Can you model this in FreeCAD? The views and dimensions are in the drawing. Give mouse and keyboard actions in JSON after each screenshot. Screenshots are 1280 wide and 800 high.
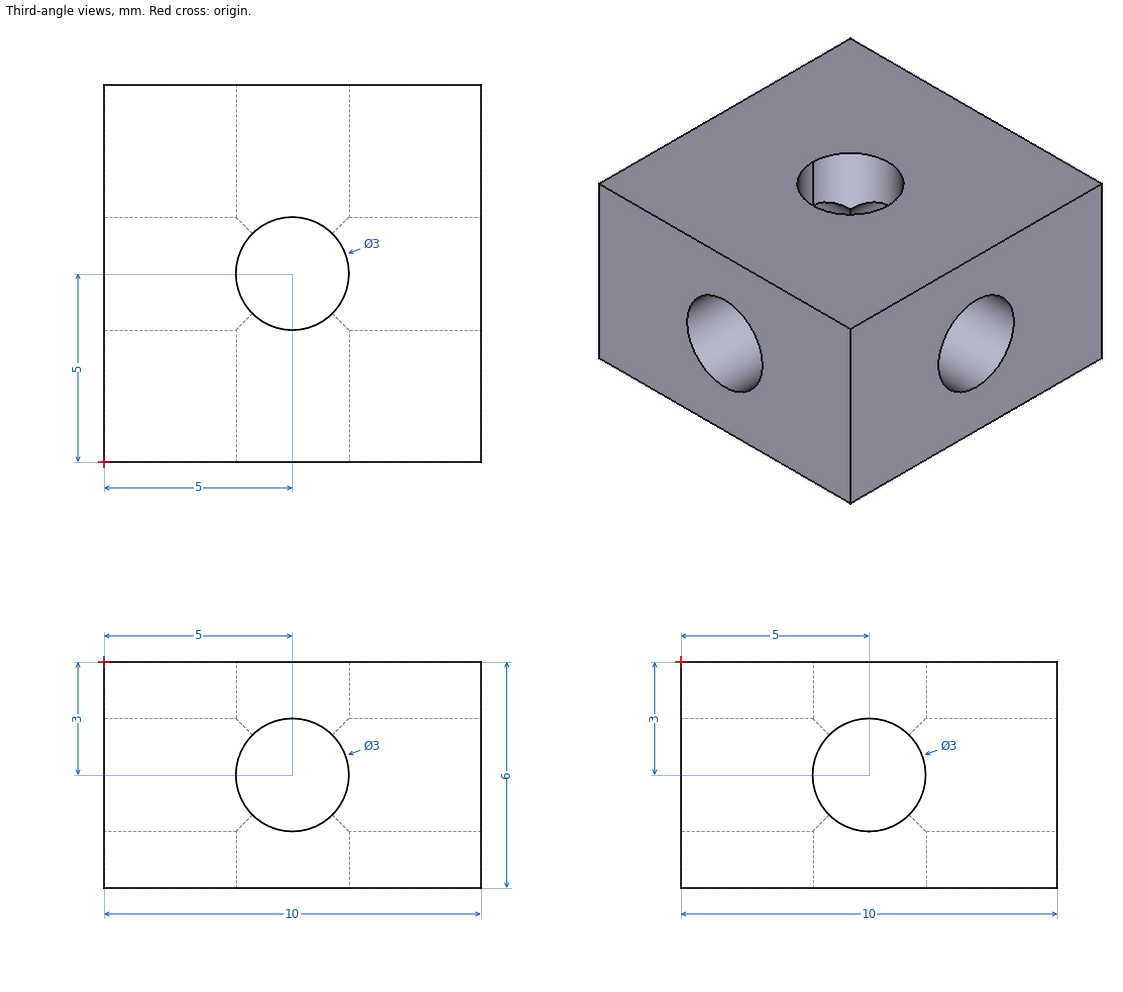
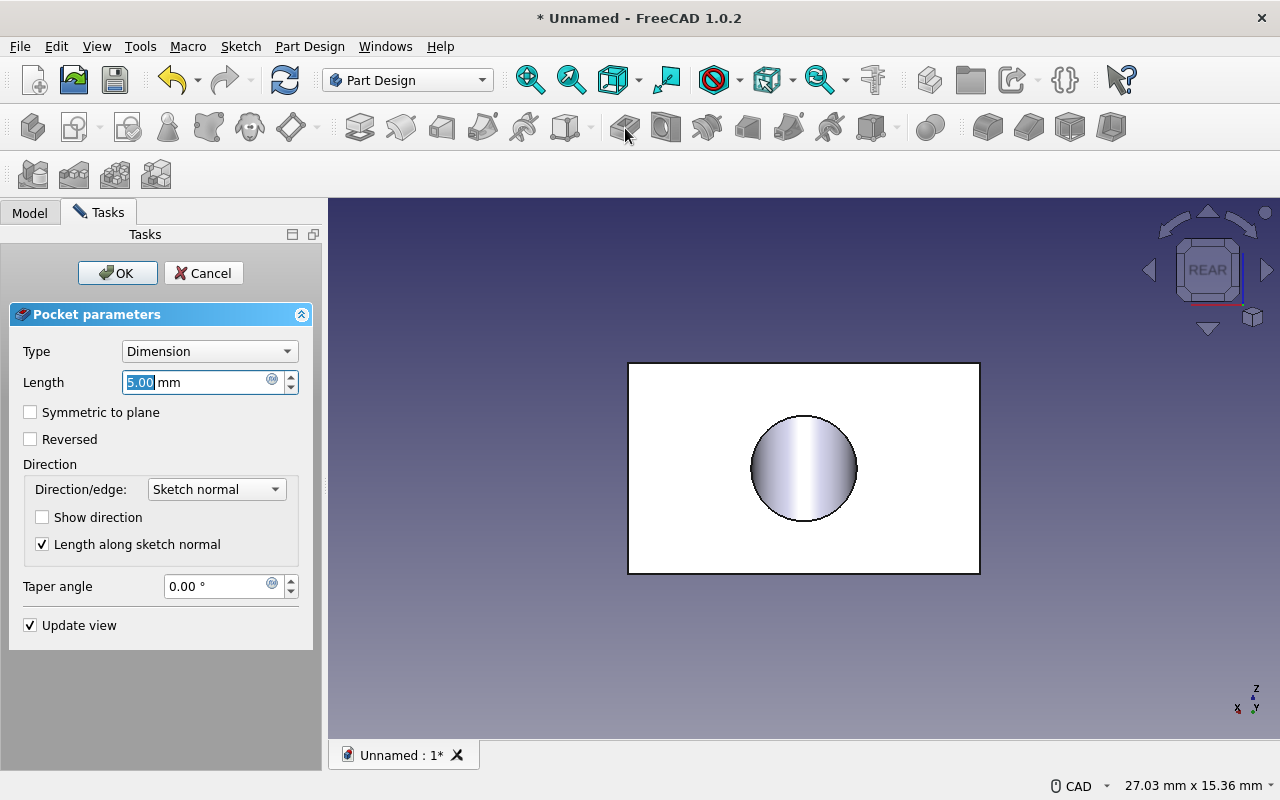
{"action": "left_click", "coordinate": [210, 352]}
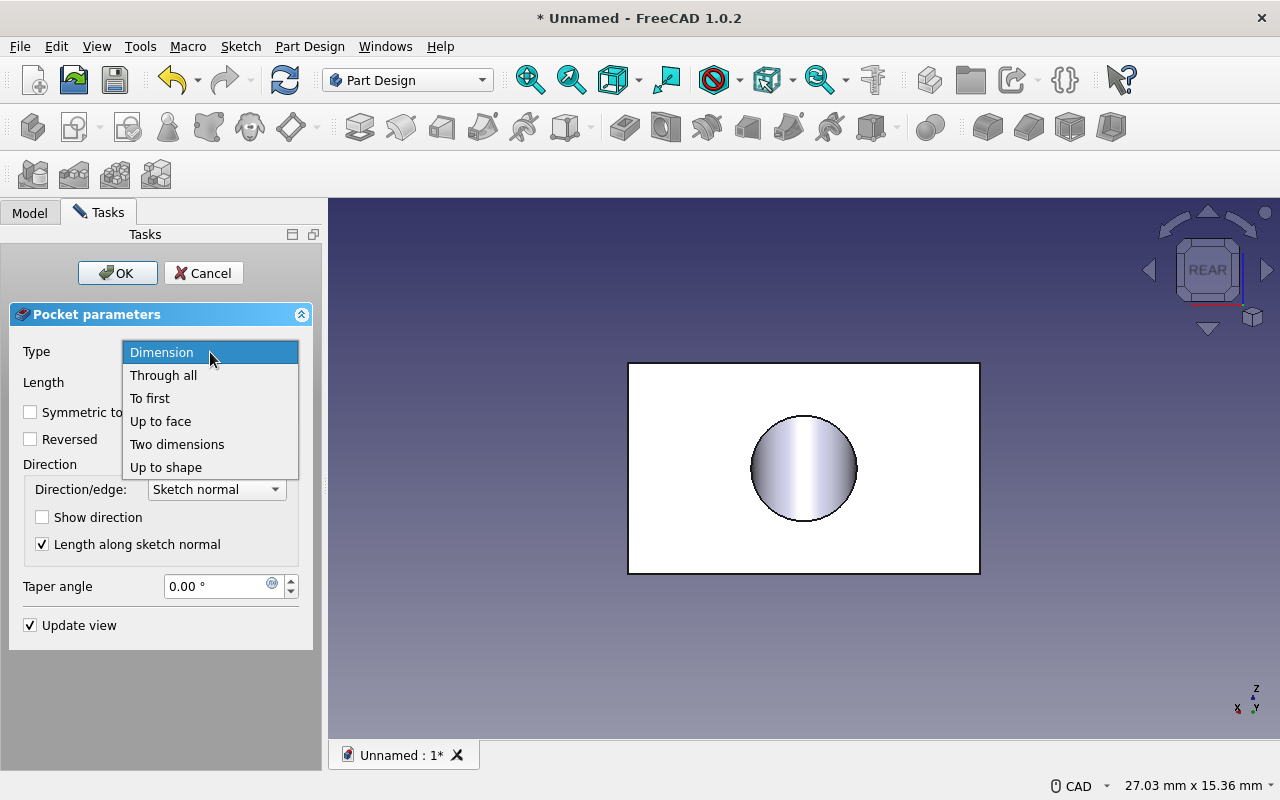
{"action": "left_click", "coordinate": [208, 376]}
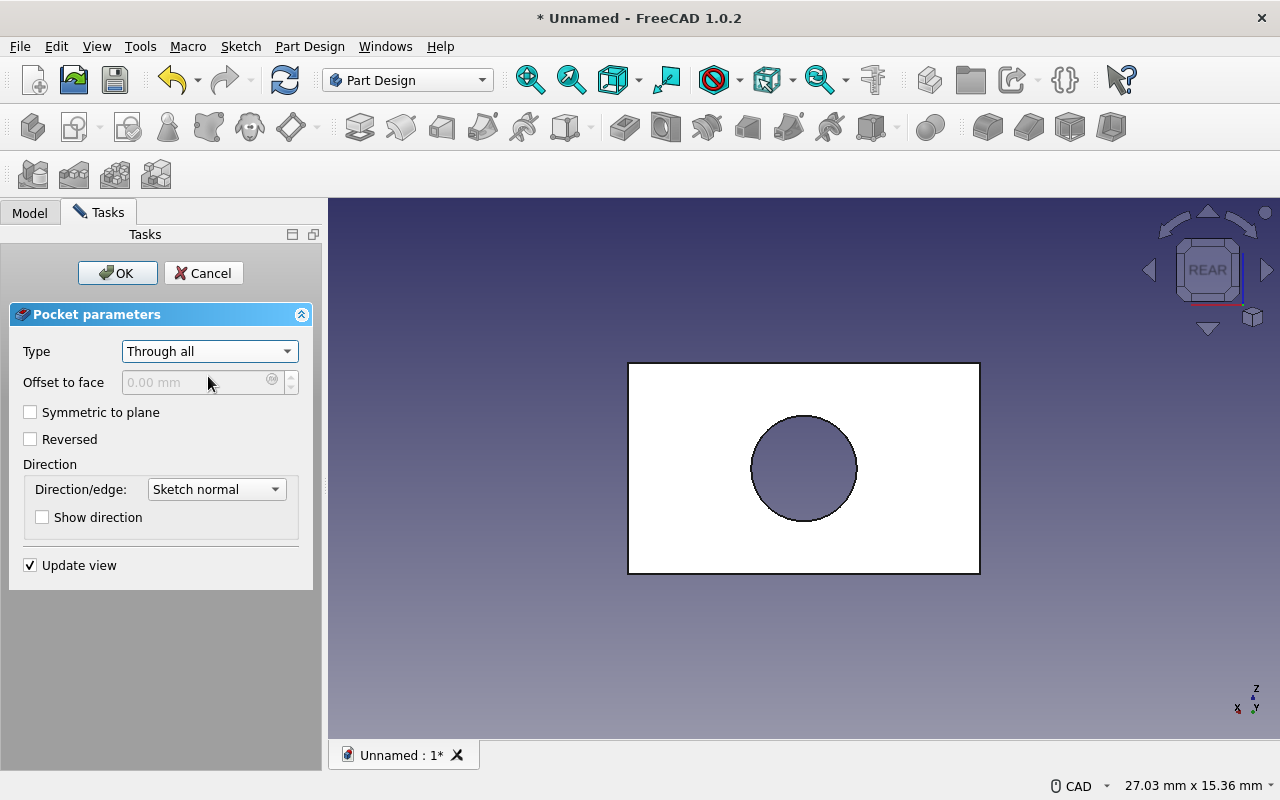
{"action": "left_click", "coordinate": [118, 273]}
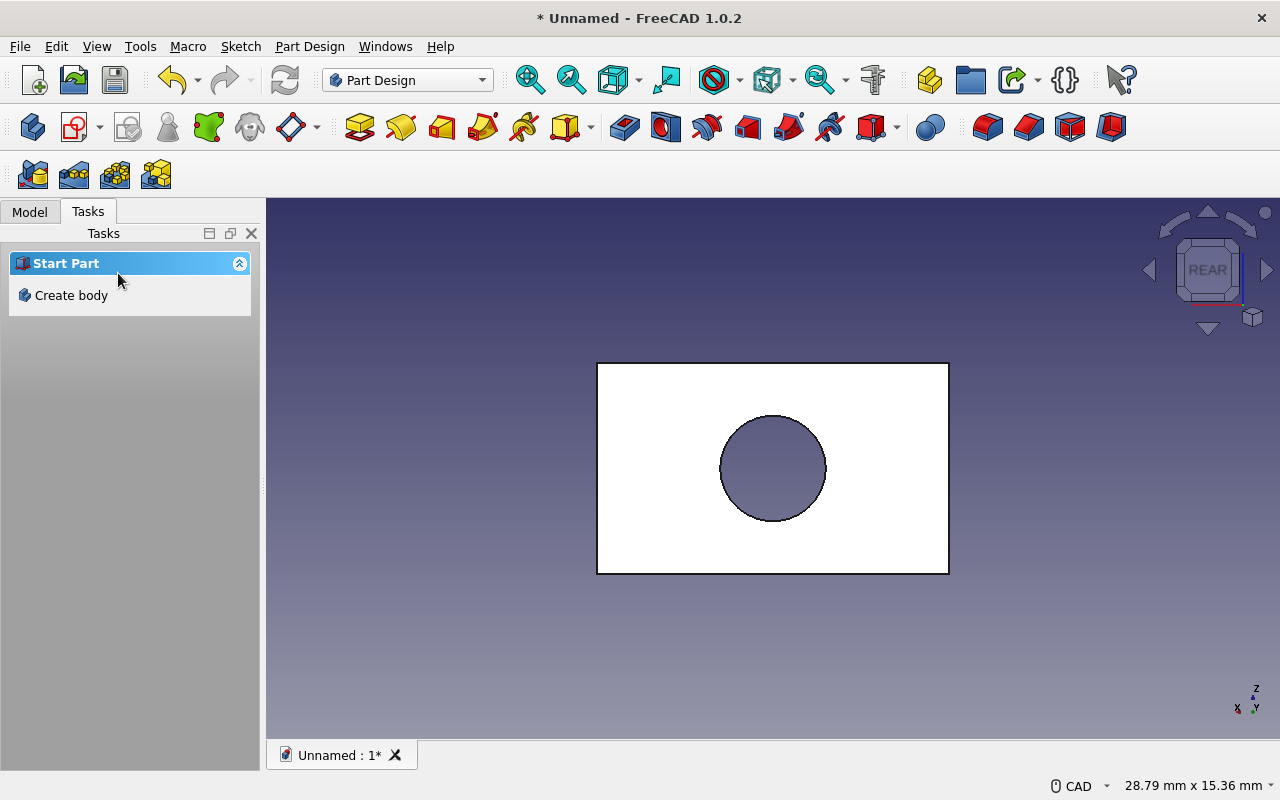
{"action": "left_click", "coordinate": [531, 80]}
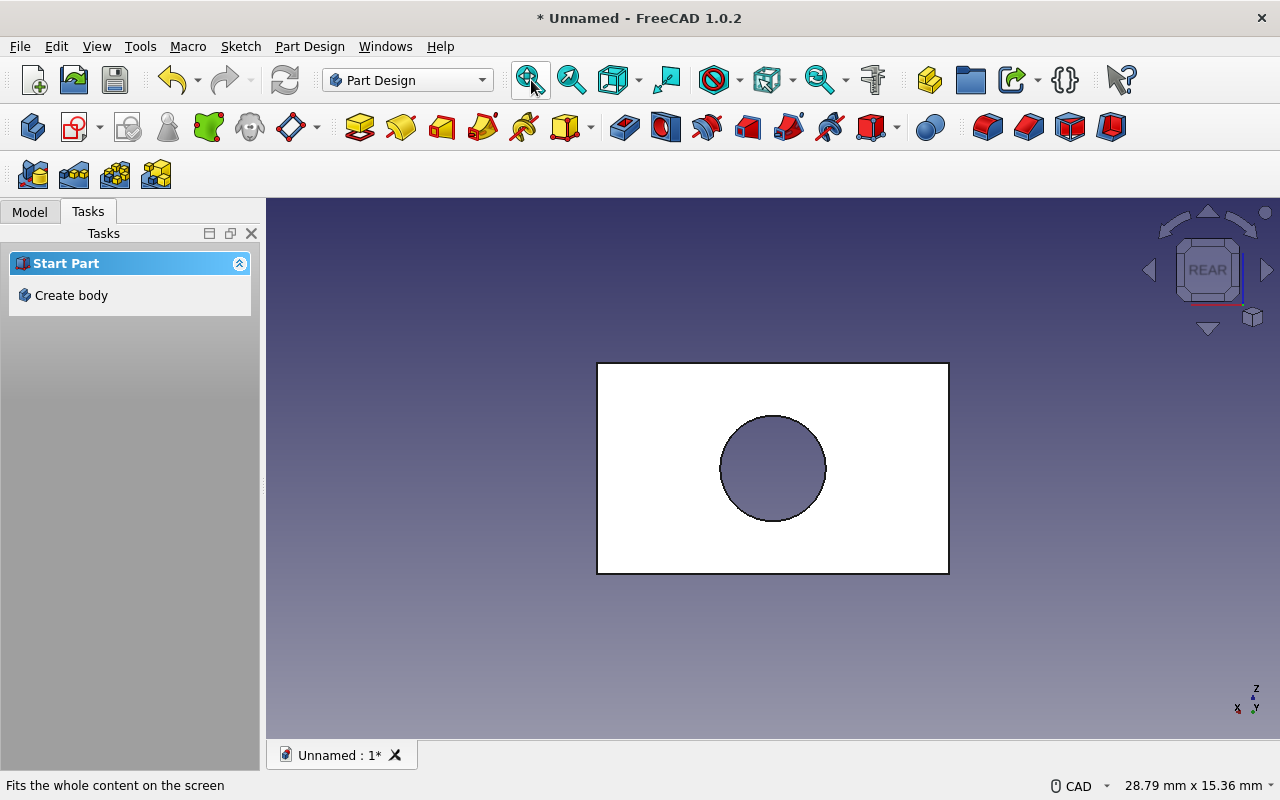
{"action": "key", "text": "0"}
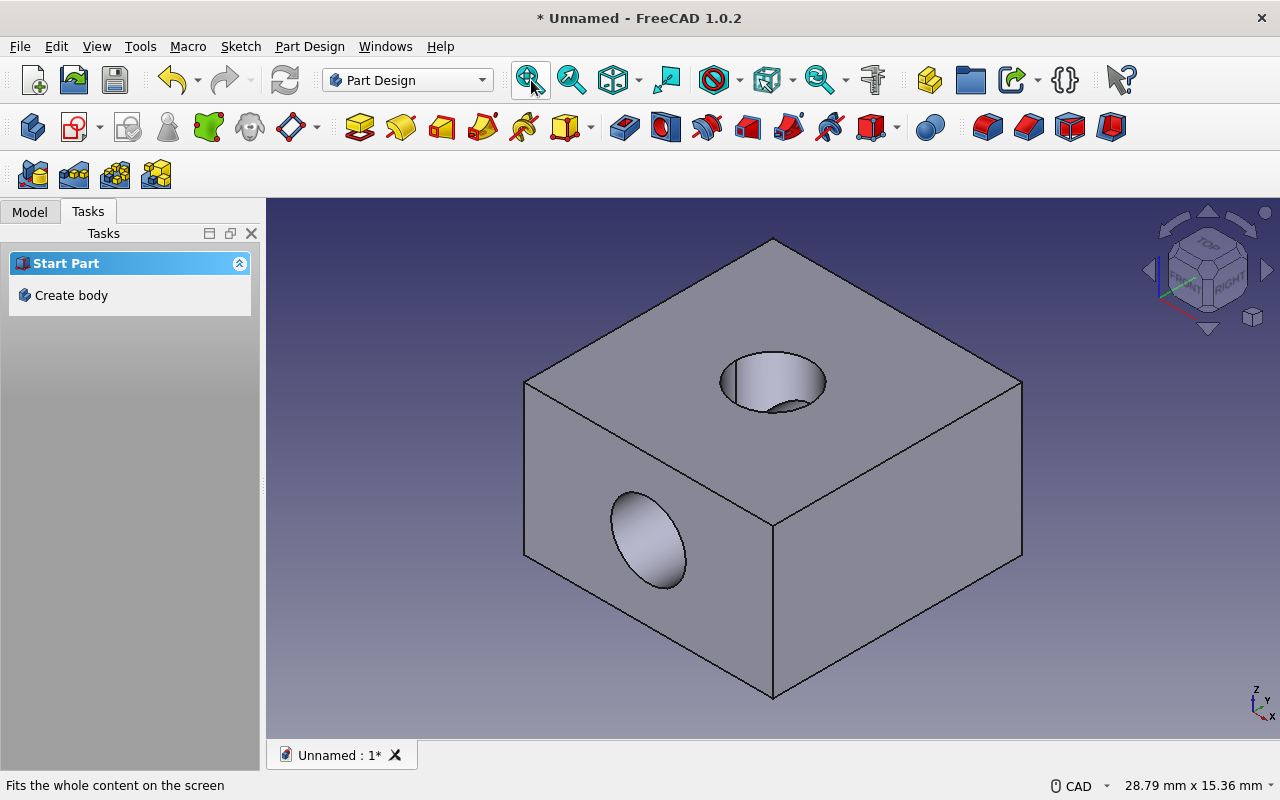
{"action": "left_click", "coordinate": [933, 519]}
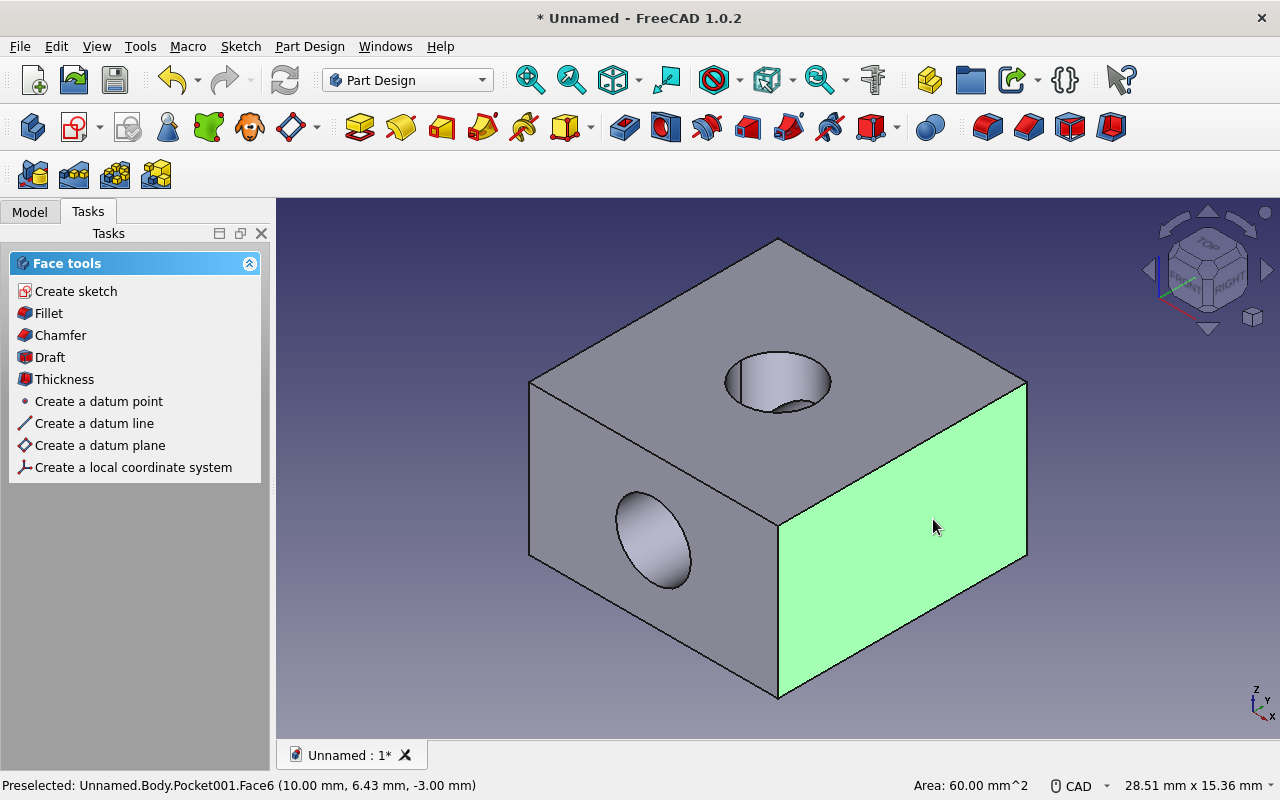
{"action": "left_click", "coordinate": [74, 128]}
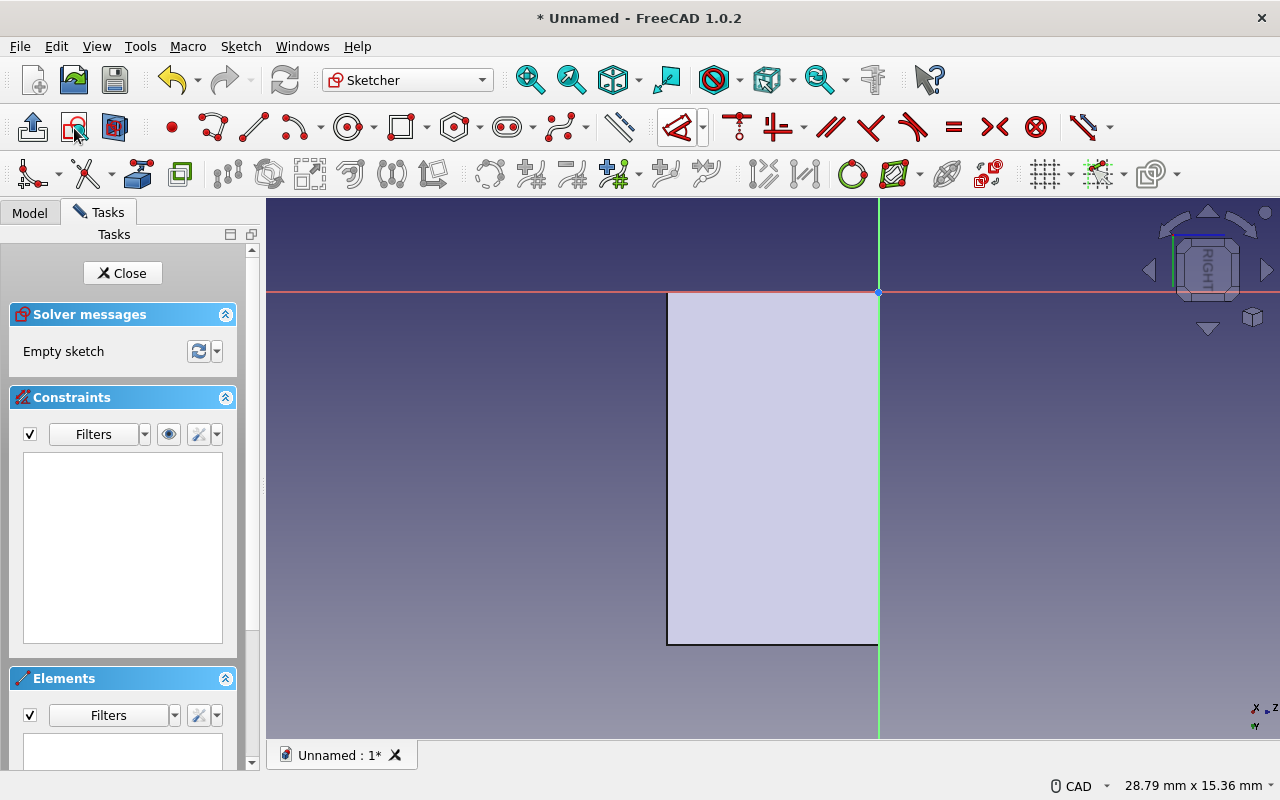
{"action": "scroll", "coordinate": [992, 282], "scroll_direction": "up", "scroll_amount": 2}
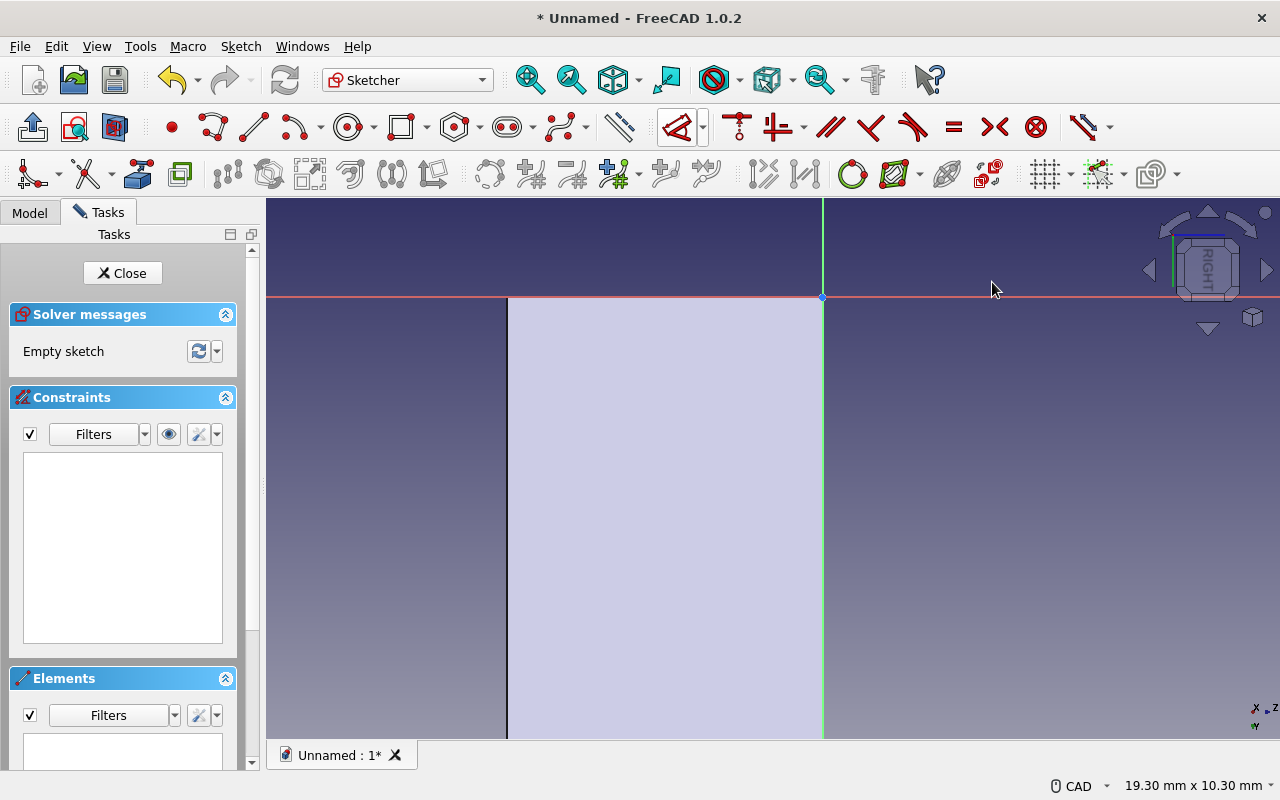
{"action": "left_click", "coordinate": [348, 128]}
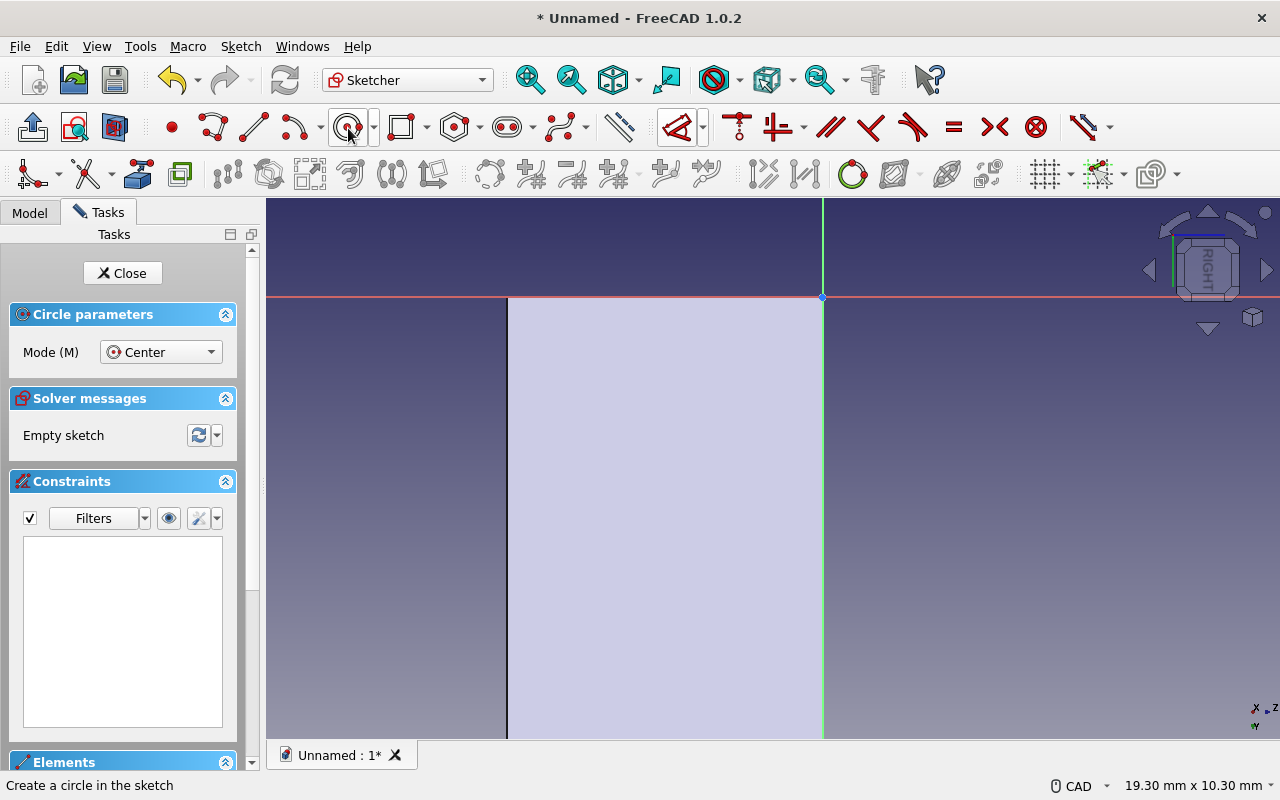
{"action": "left_click", "coordinate": [665, 560]}
{"action": "mouse_move", "coordinate": [721, 504]}